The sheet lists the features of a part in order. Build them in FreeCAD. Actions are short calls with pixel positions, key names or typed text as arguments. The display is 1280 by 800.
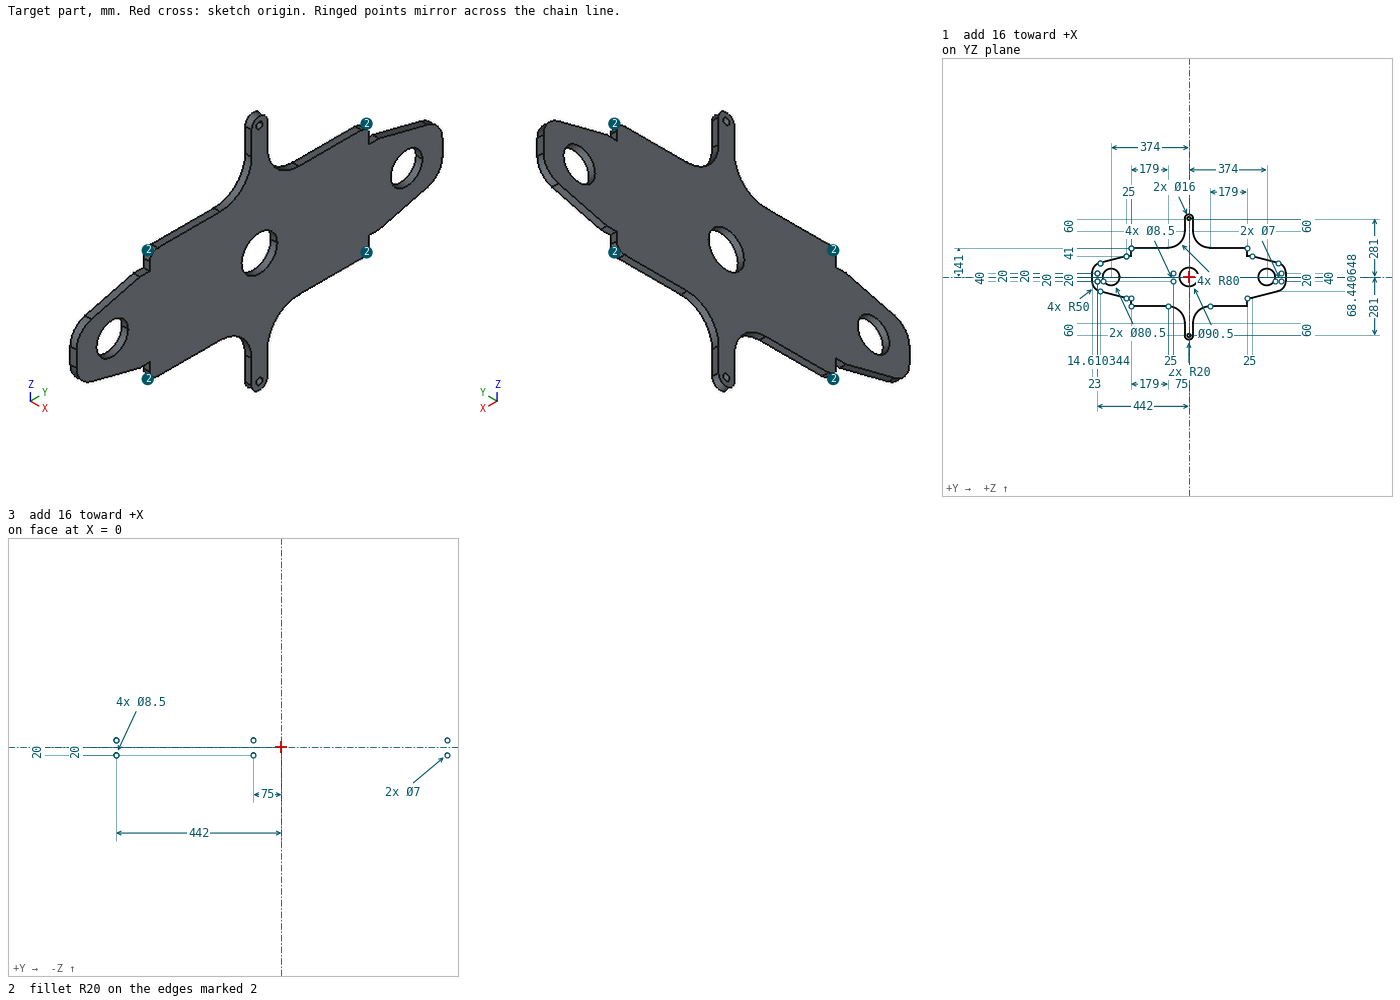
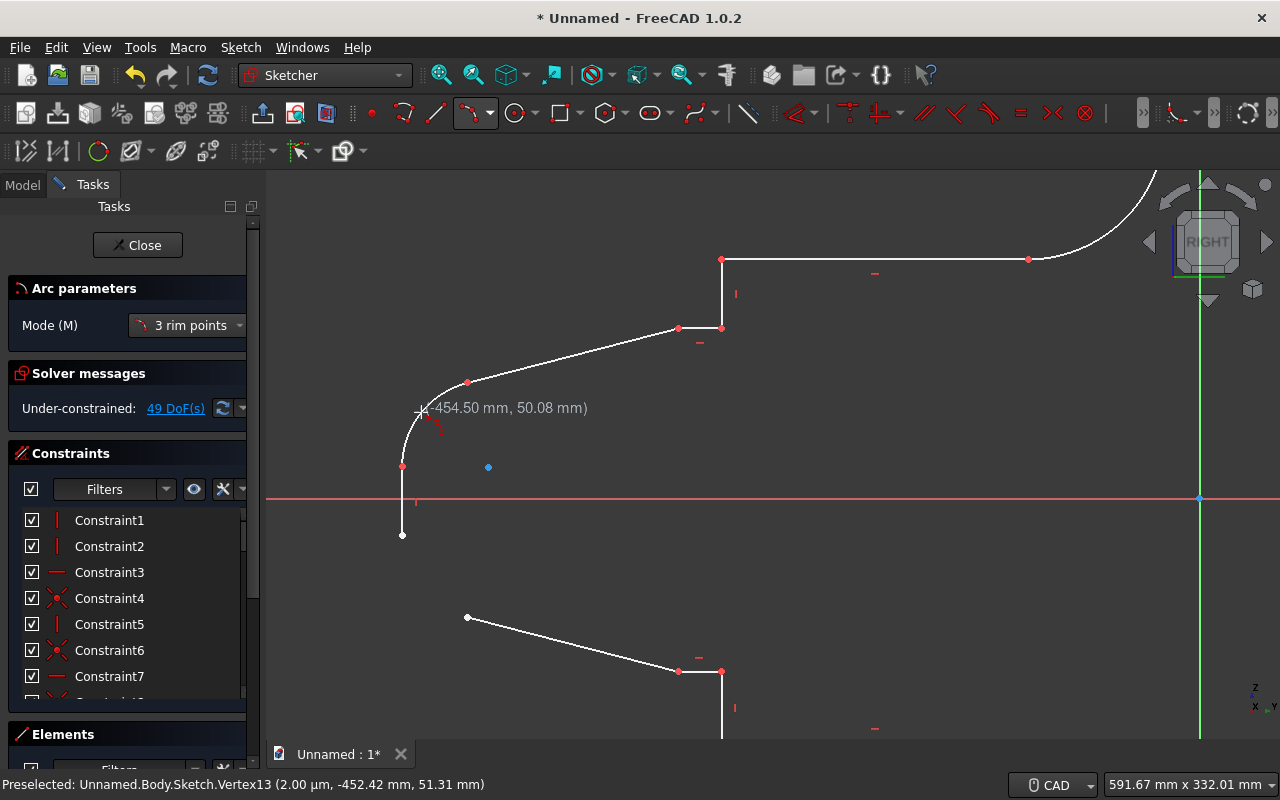
click(402, 536)
click(467, 617)
click(421, 586)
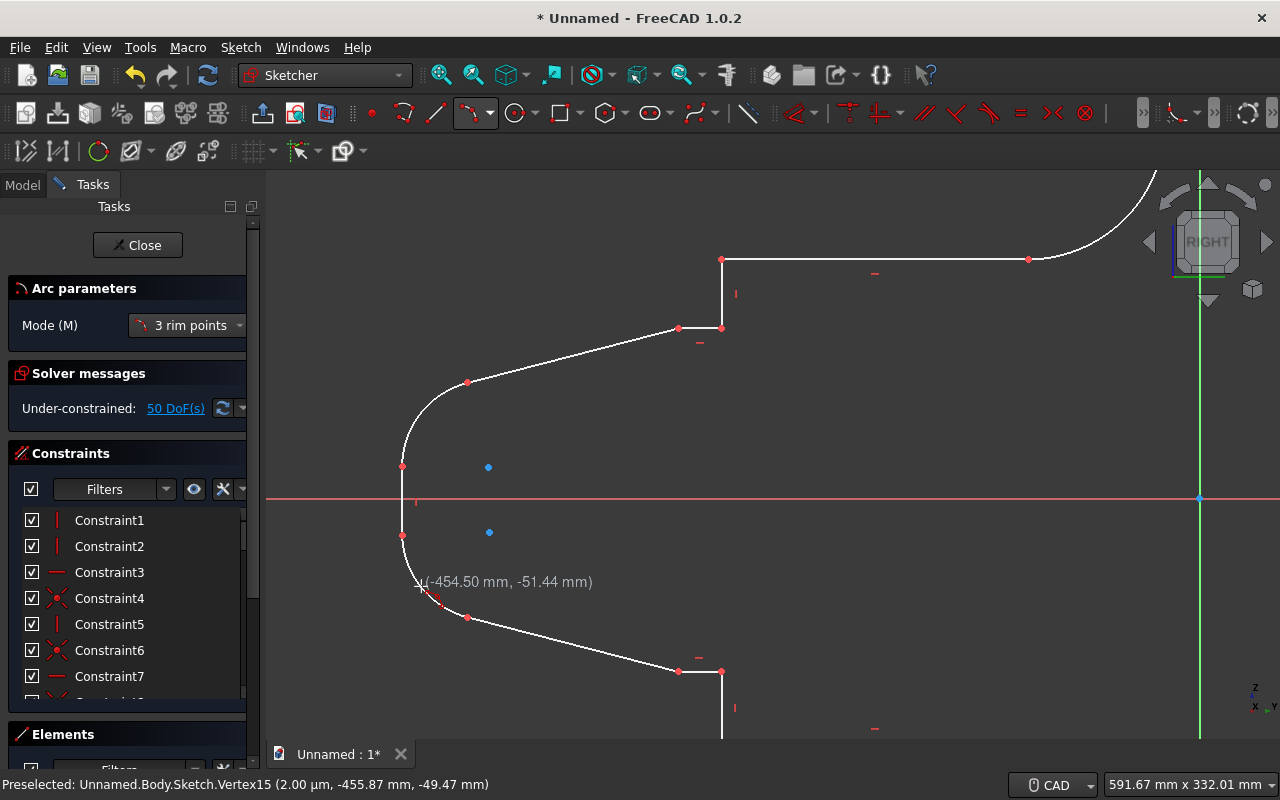
scroll(416, 429, down, 5)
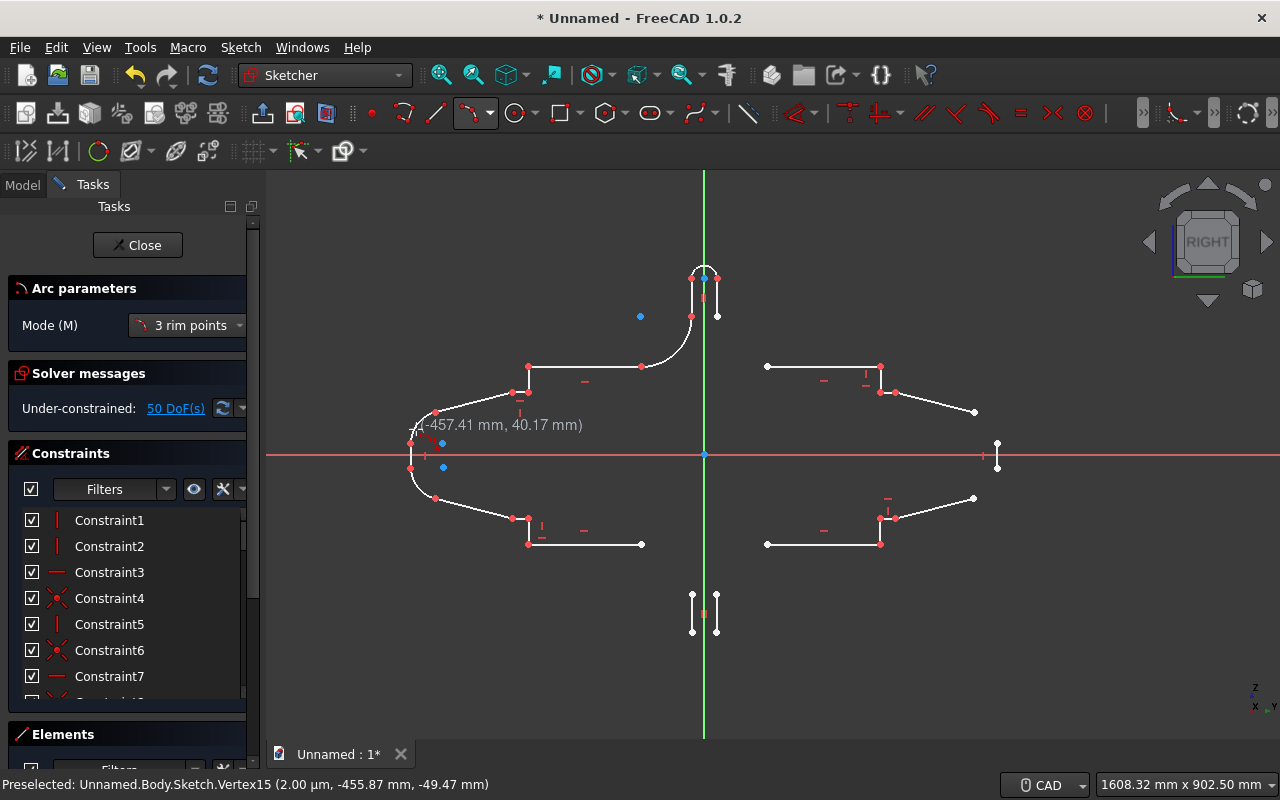
click(641, 545)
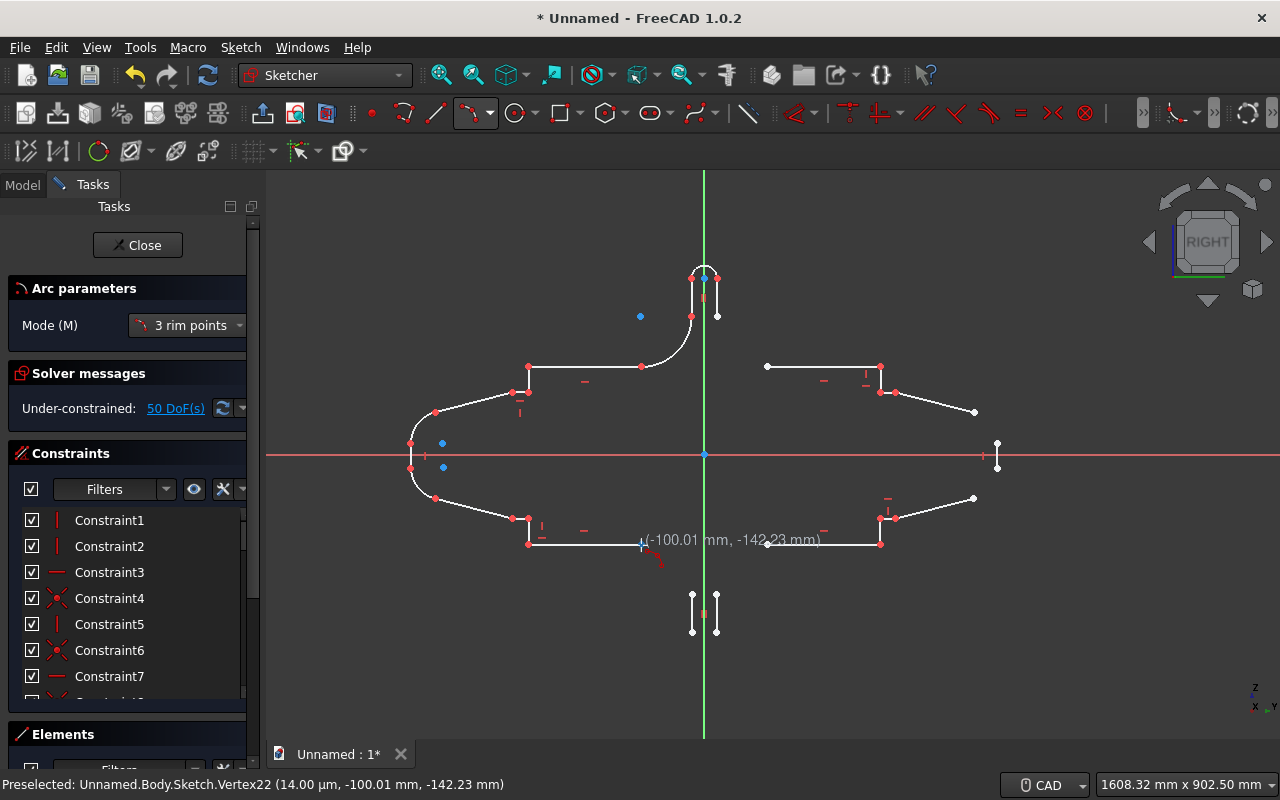
scroll(692, 594, up, 2)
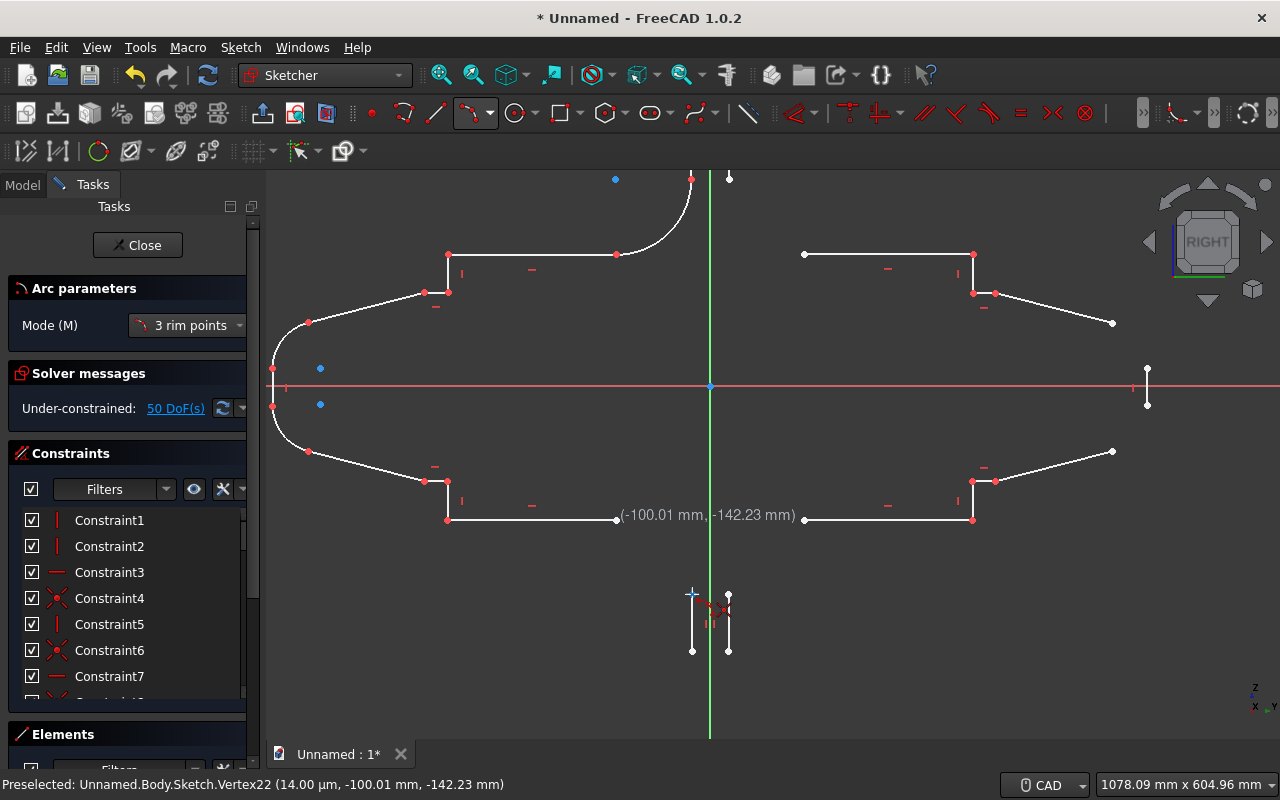
click(692, 595)
click(670, 541)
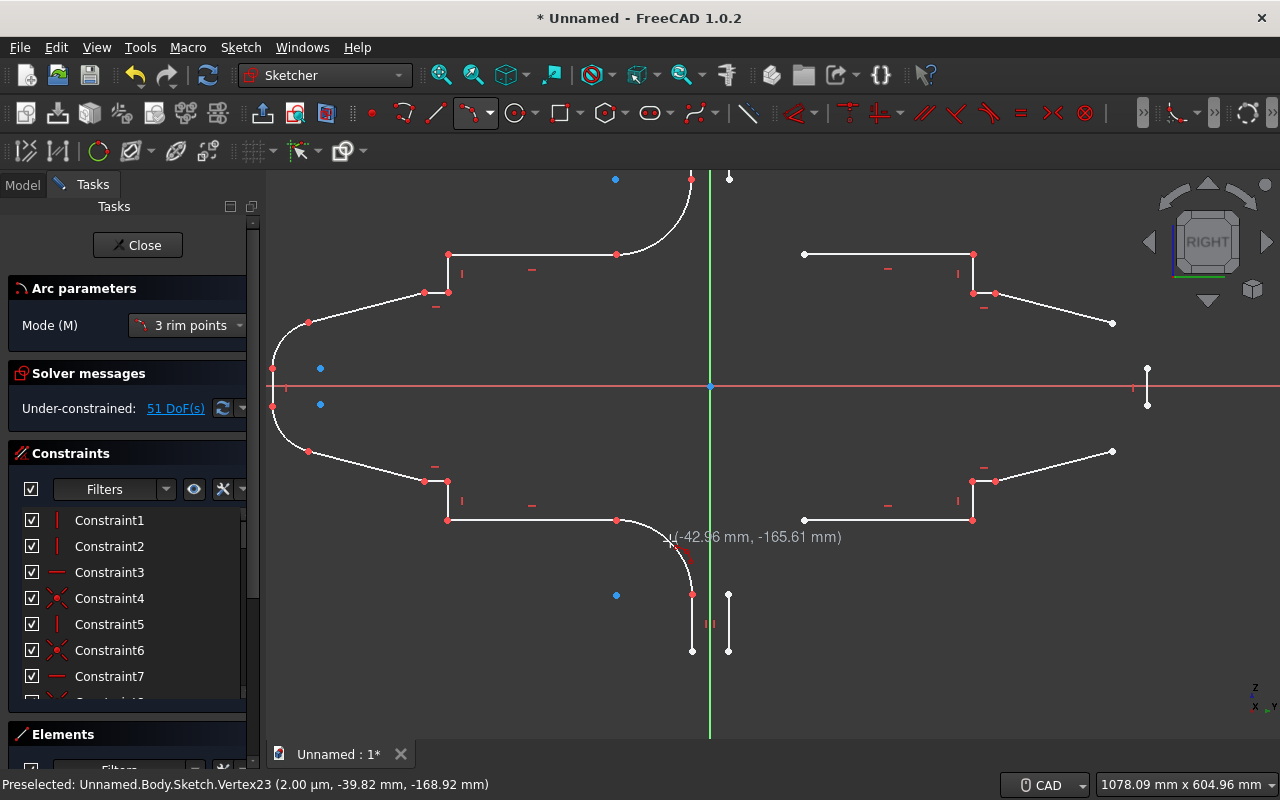
click(692, 652)
click(729, 652)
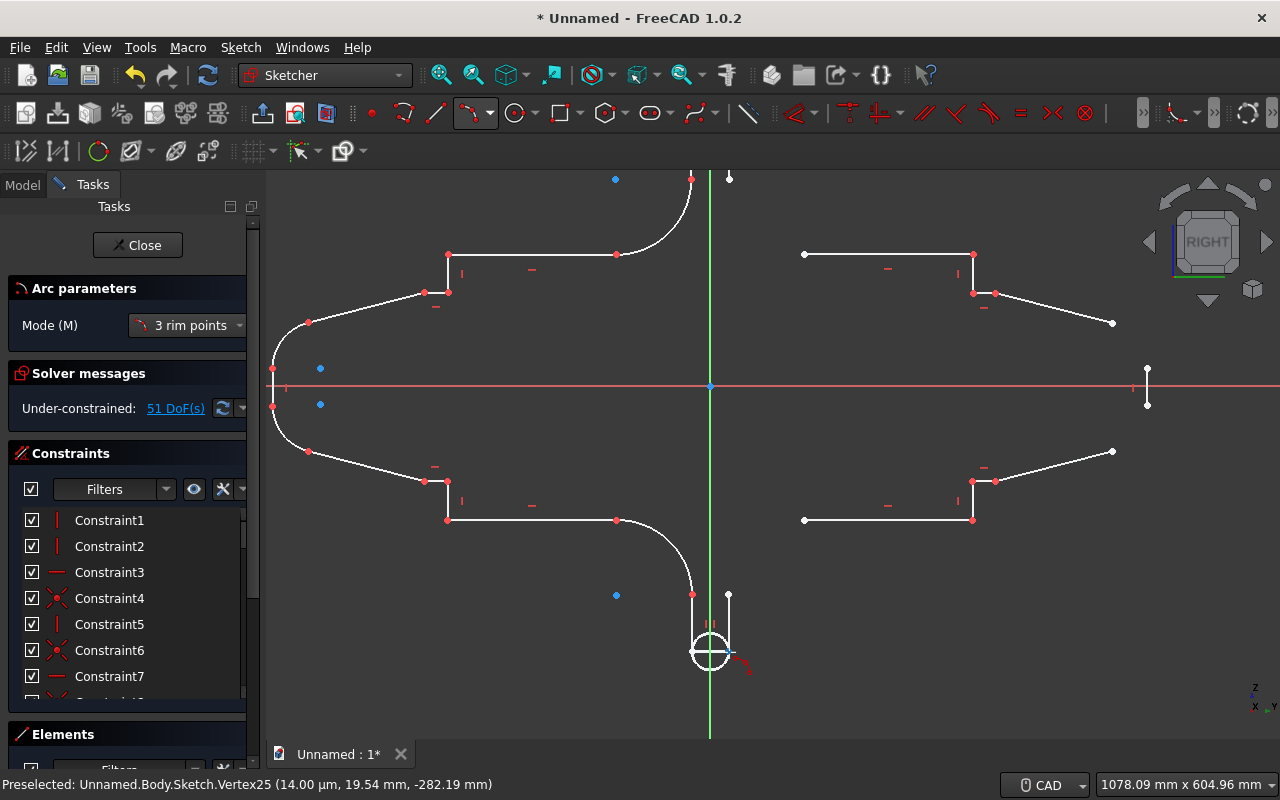
scroll(699, 666, up, 2)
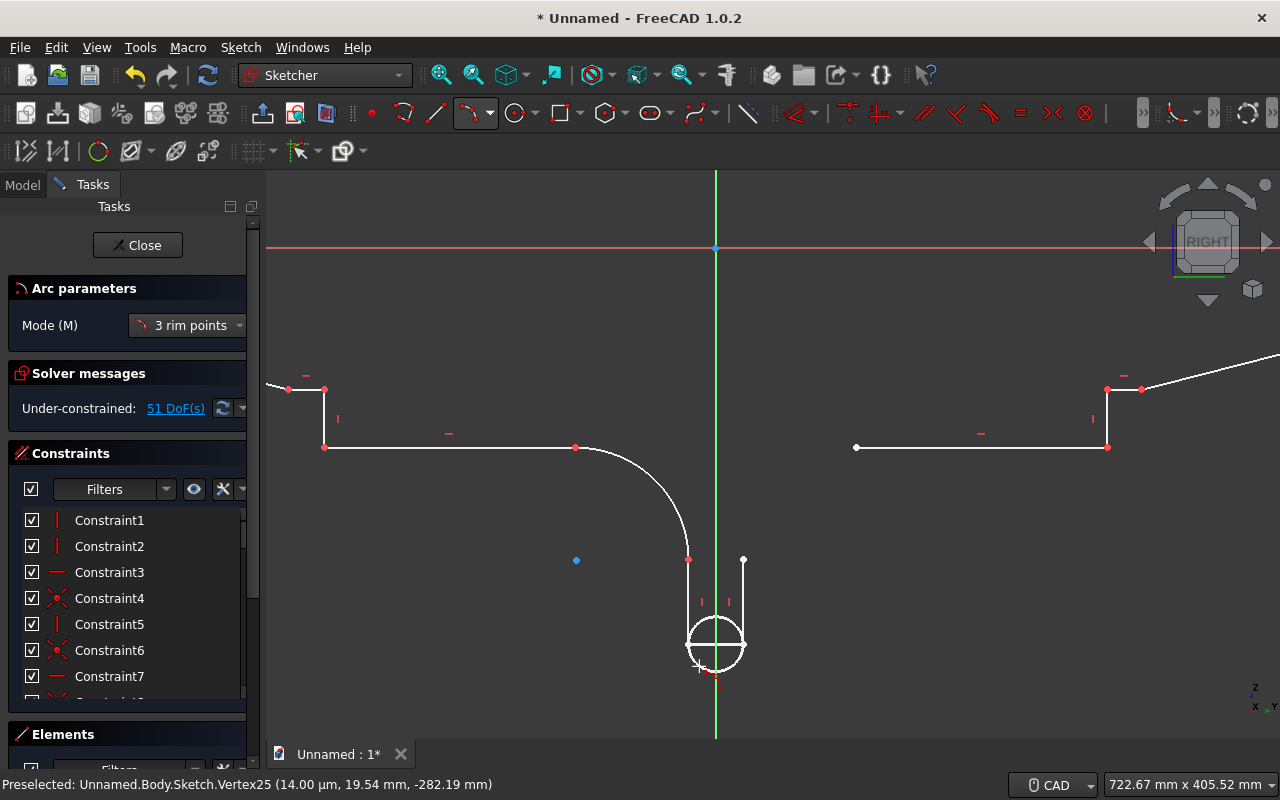
click(699, 665)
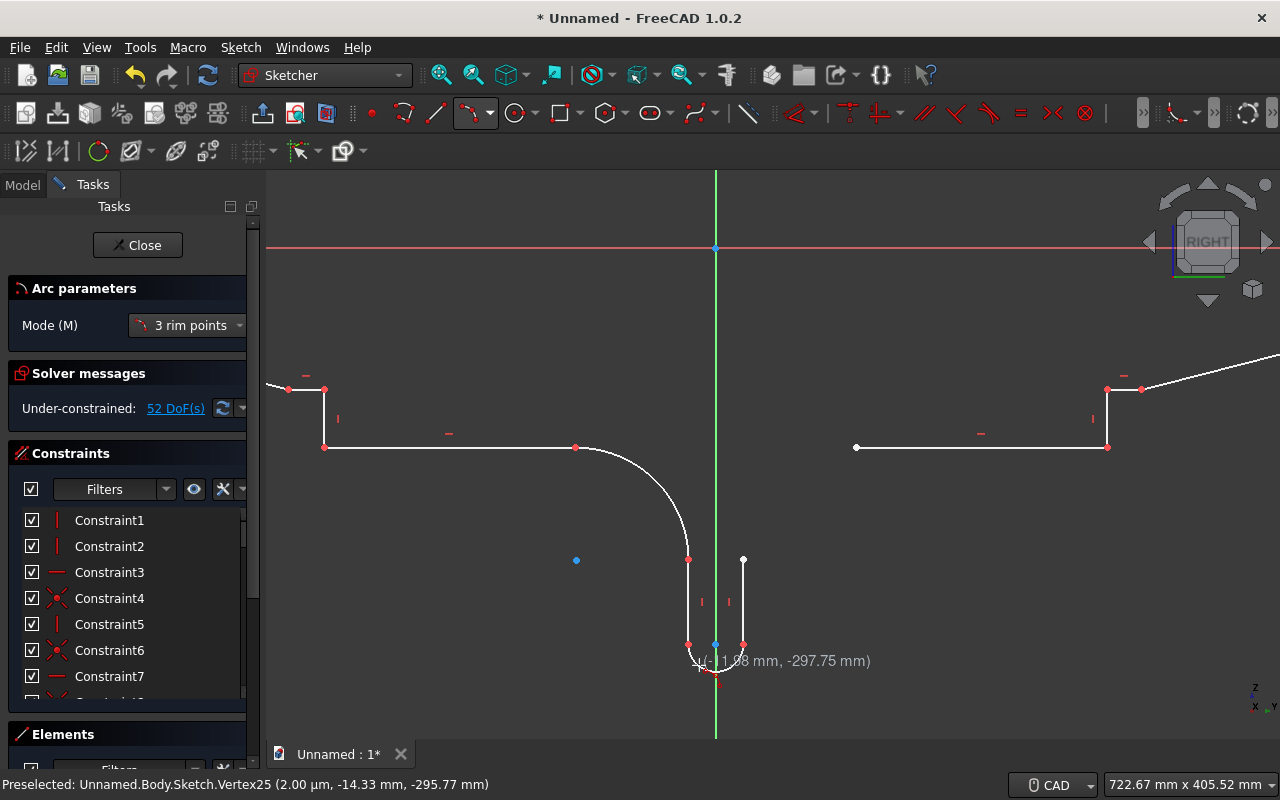
click(743, 559)
click(856, 448)
click(777, 479)